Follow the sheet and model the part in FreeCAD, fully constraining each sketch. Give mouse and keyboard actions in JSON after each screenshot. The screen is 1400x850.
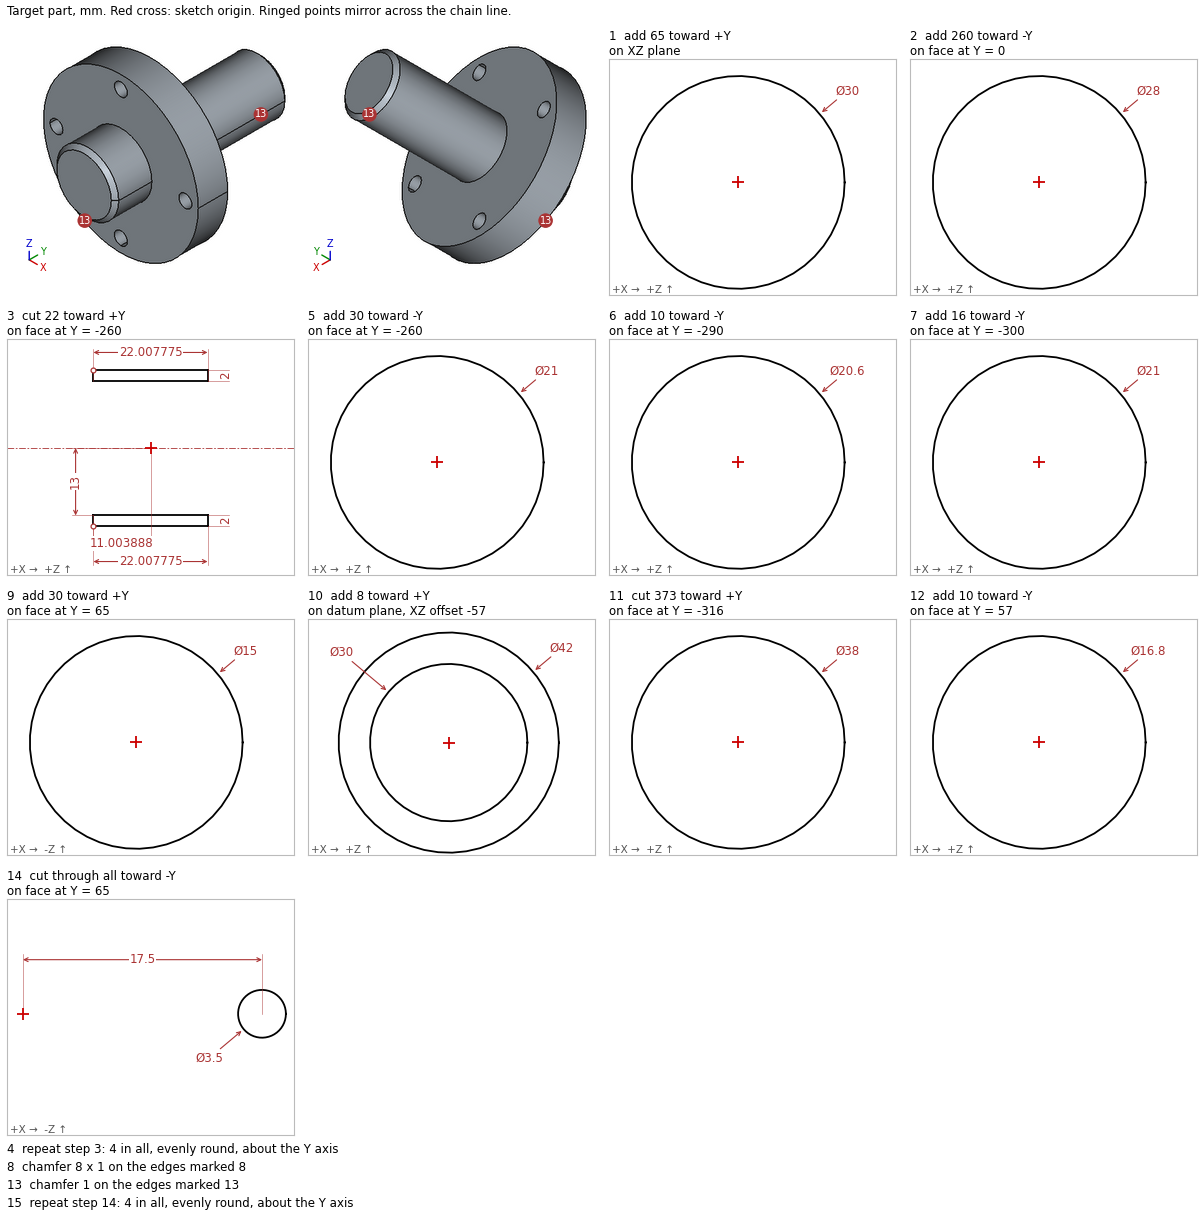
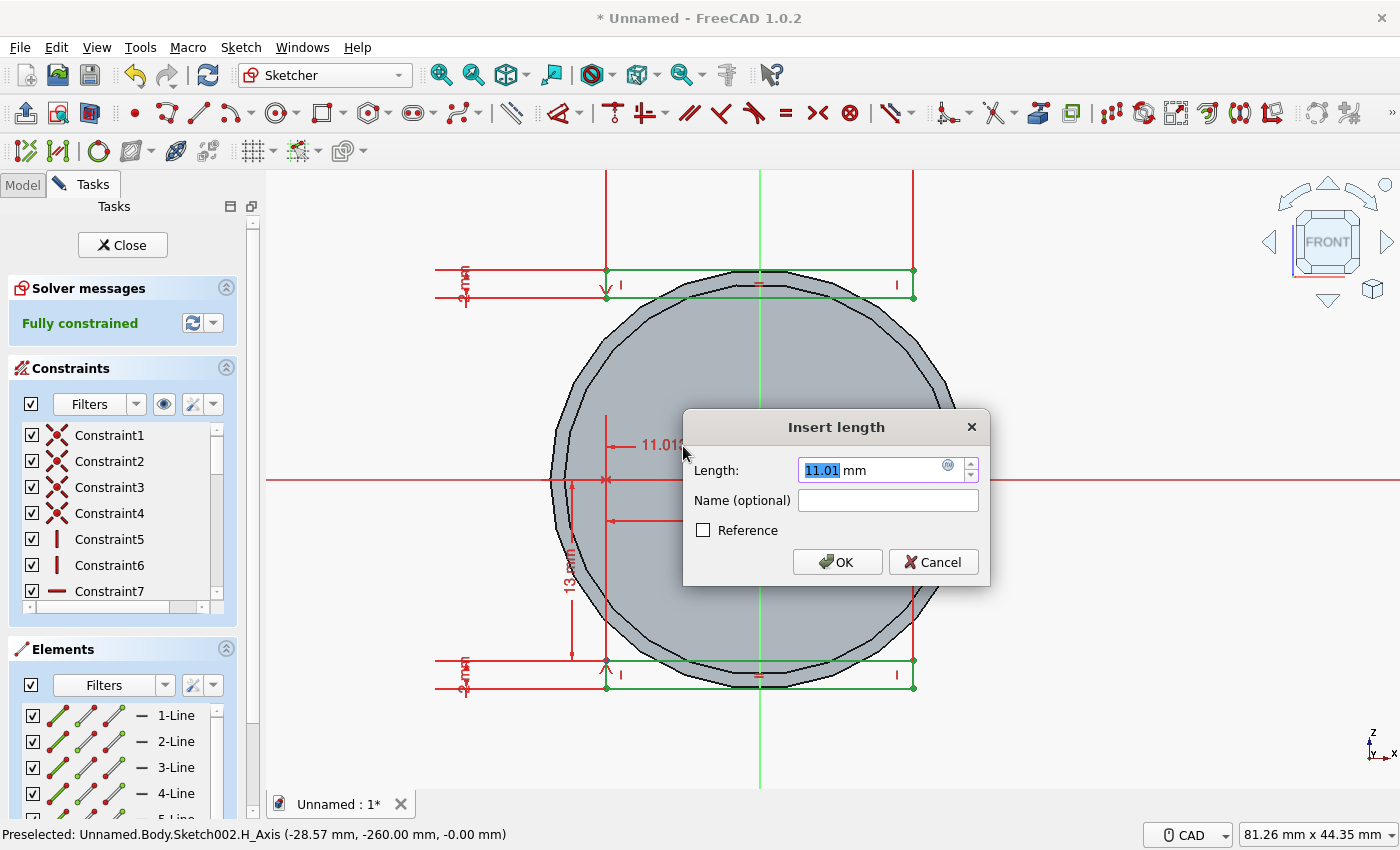
{"action": "type", "text": "11.003888"}
{"action": "key", "text": "Return"}
{"action": "key", "text": "Escape"}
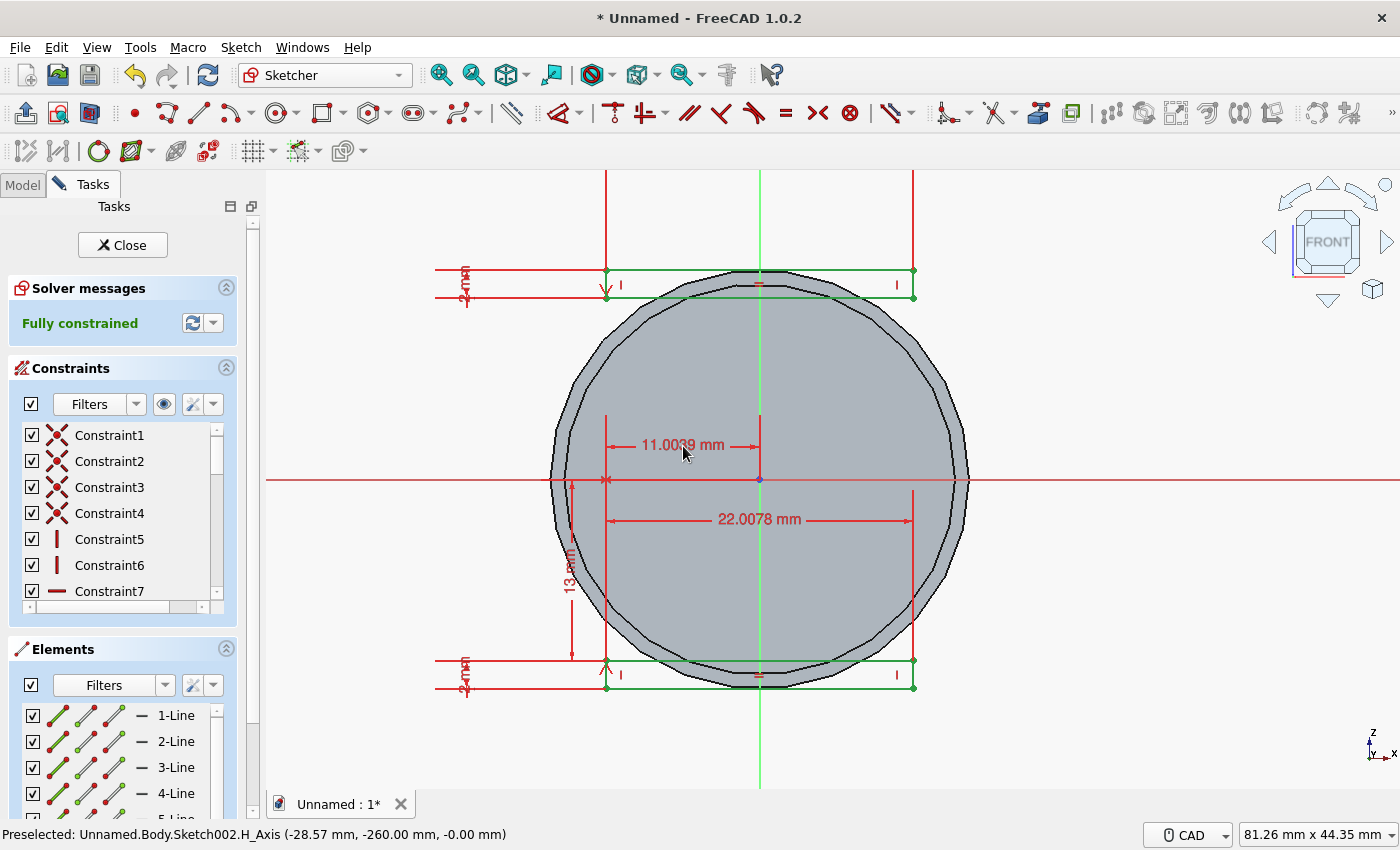
{"action": "left_click", "coordinate": [123, 245]}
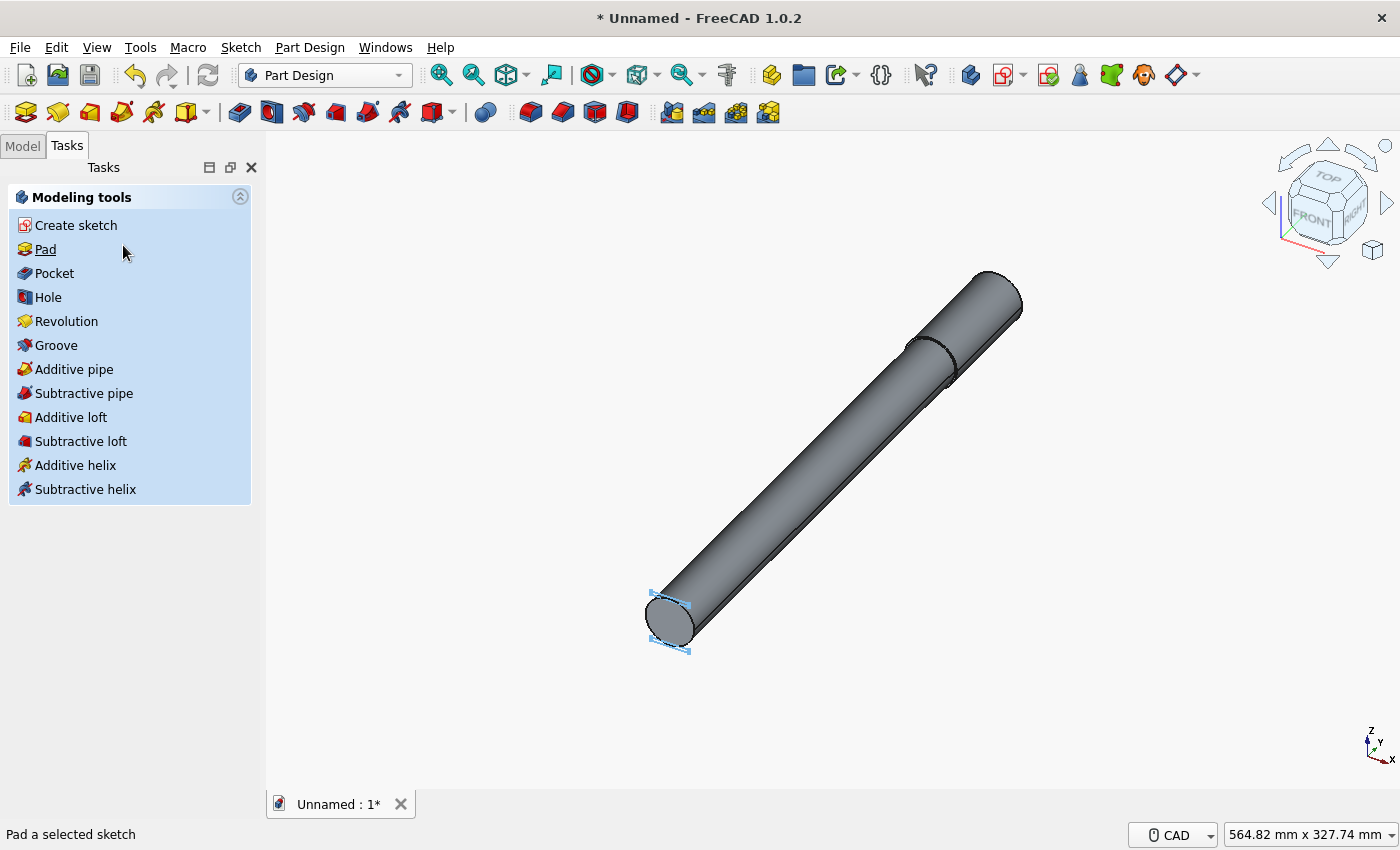
{"action": "left_click", "coordinate": [240, 112]}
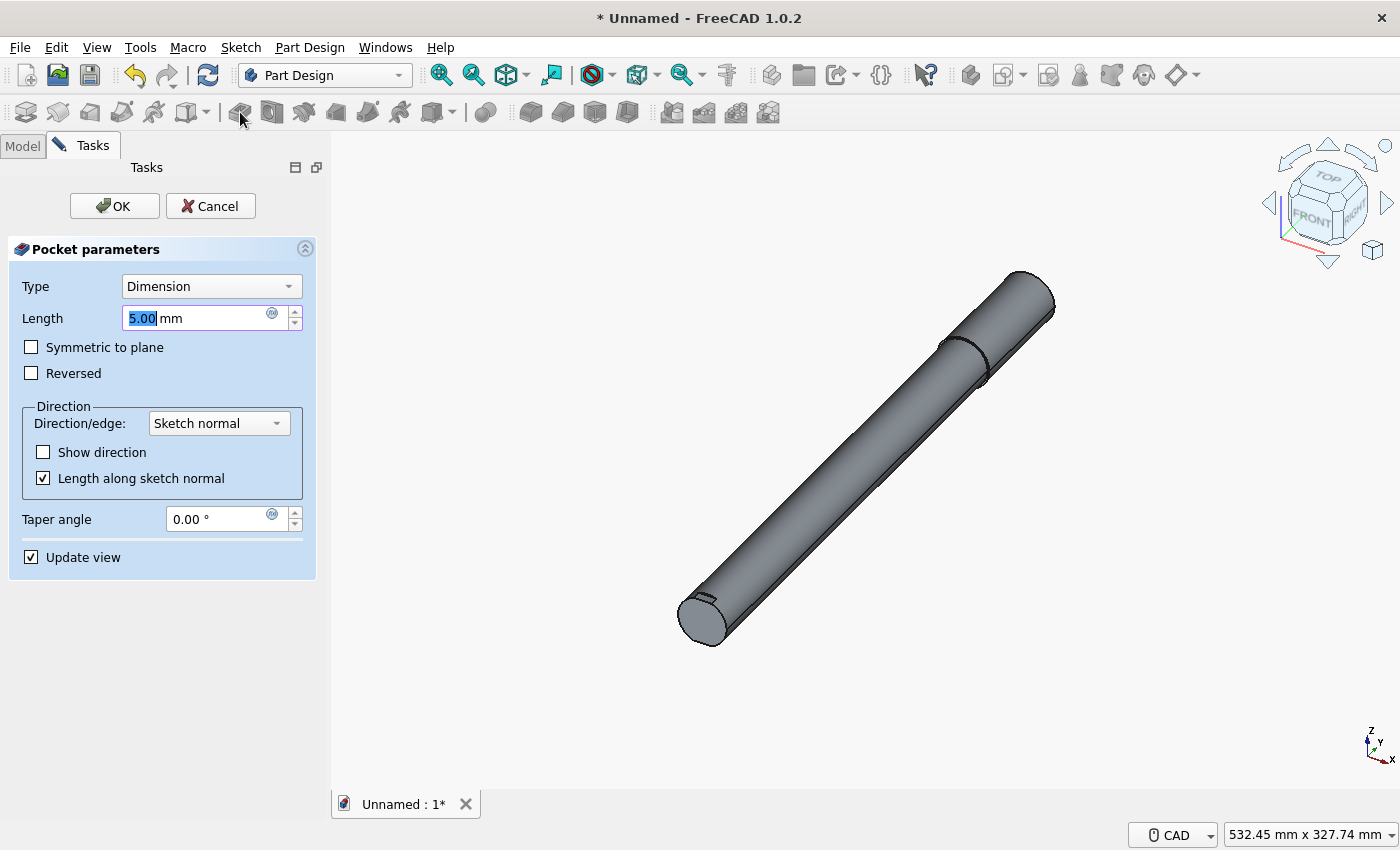
{"action": "type", "text": "22"}
{"action": "key", "text": "Tab"}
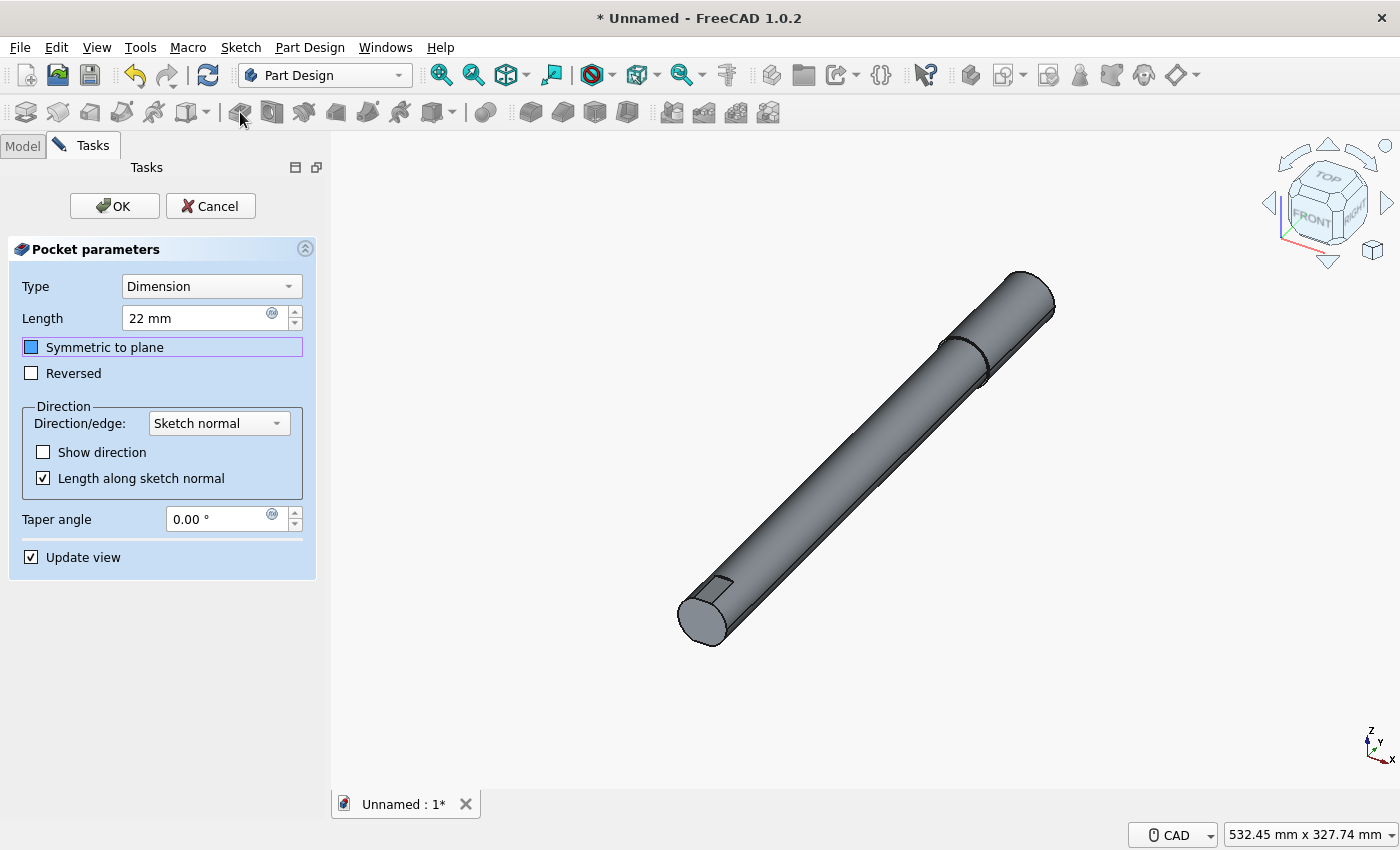
{"action": "left_click", "coordinate": [115, 206]}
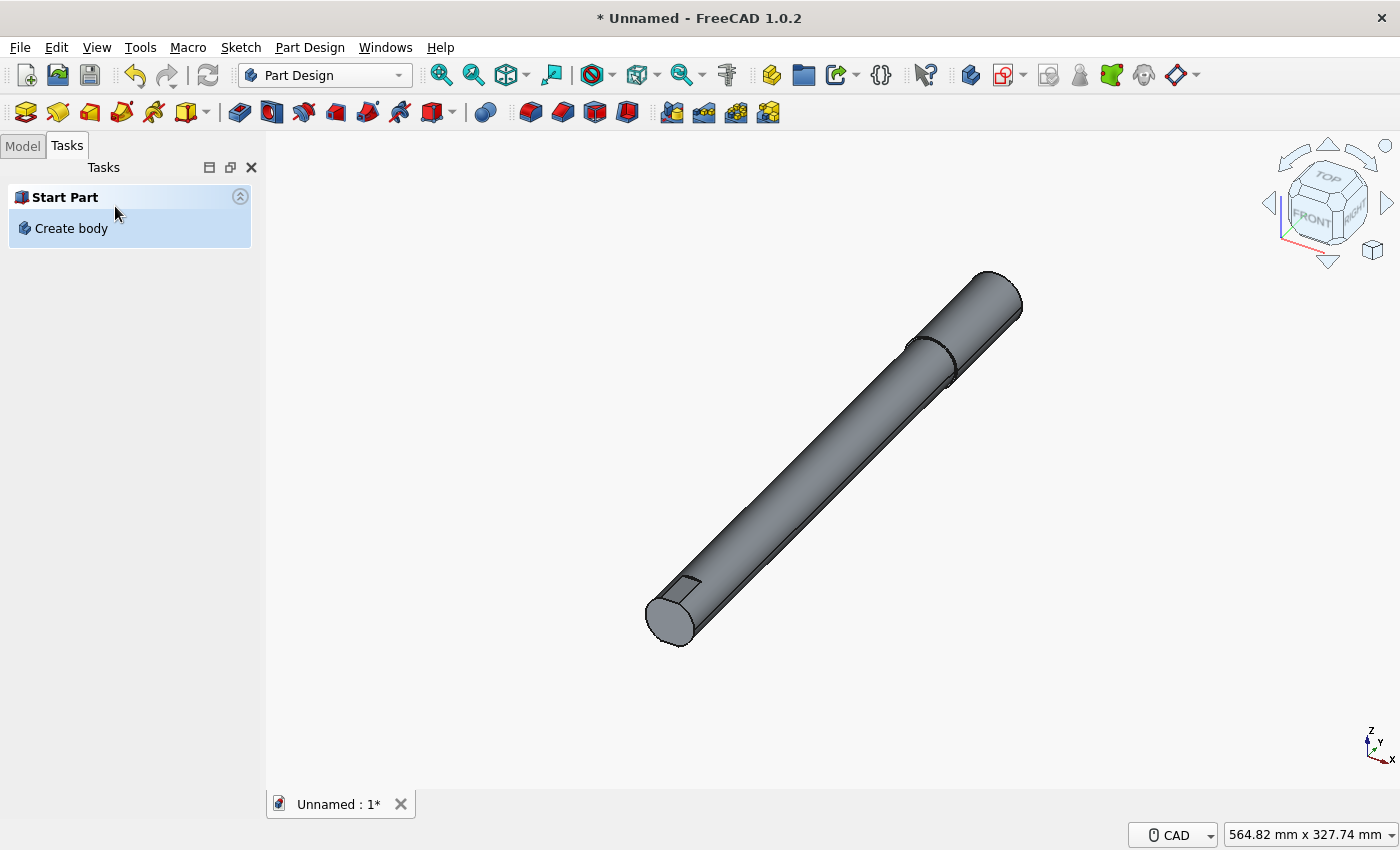
{"action": "left_click", "coordinate": [23, 145]}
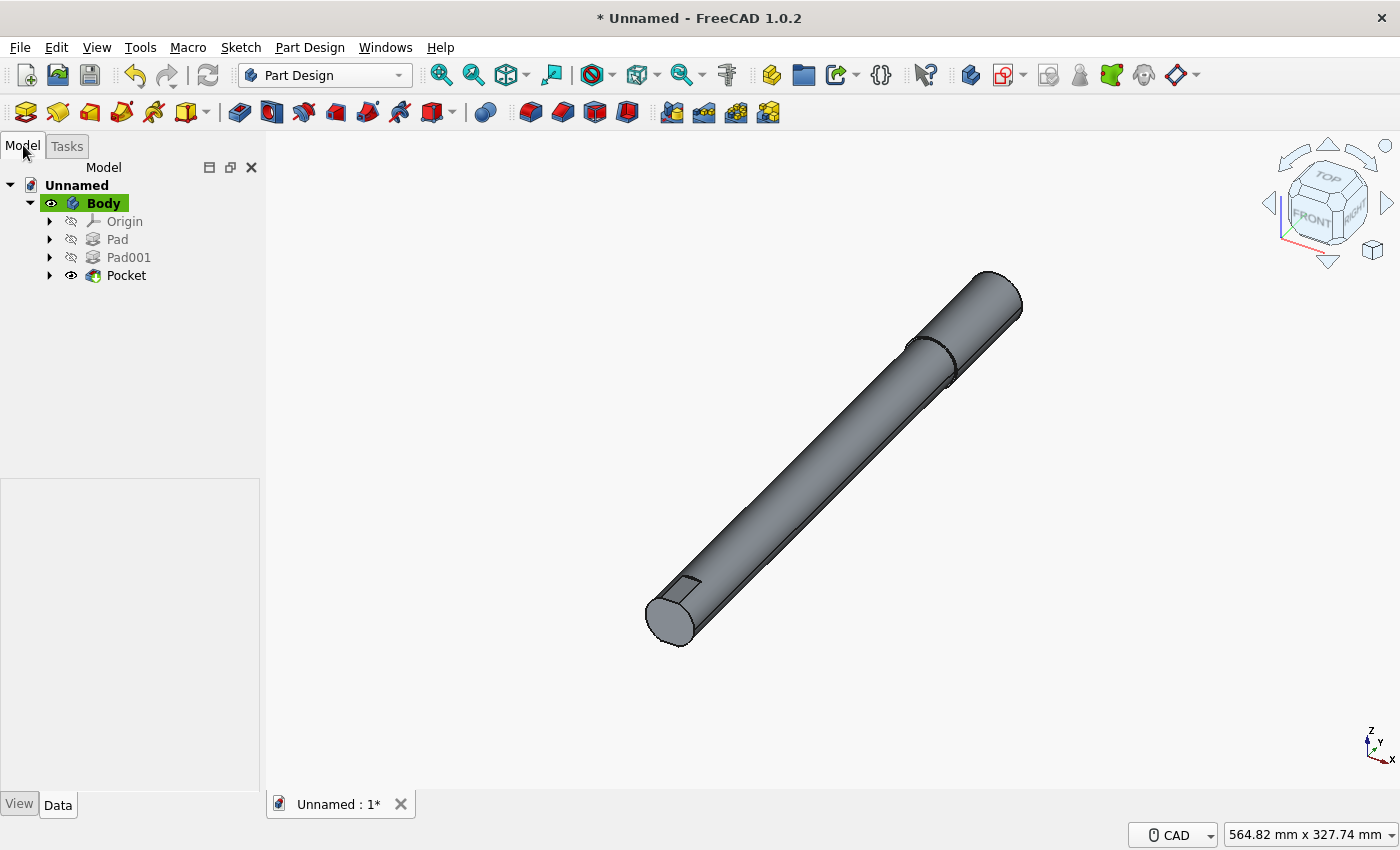
{"action": "left_click", "coordinate": [116, 275]}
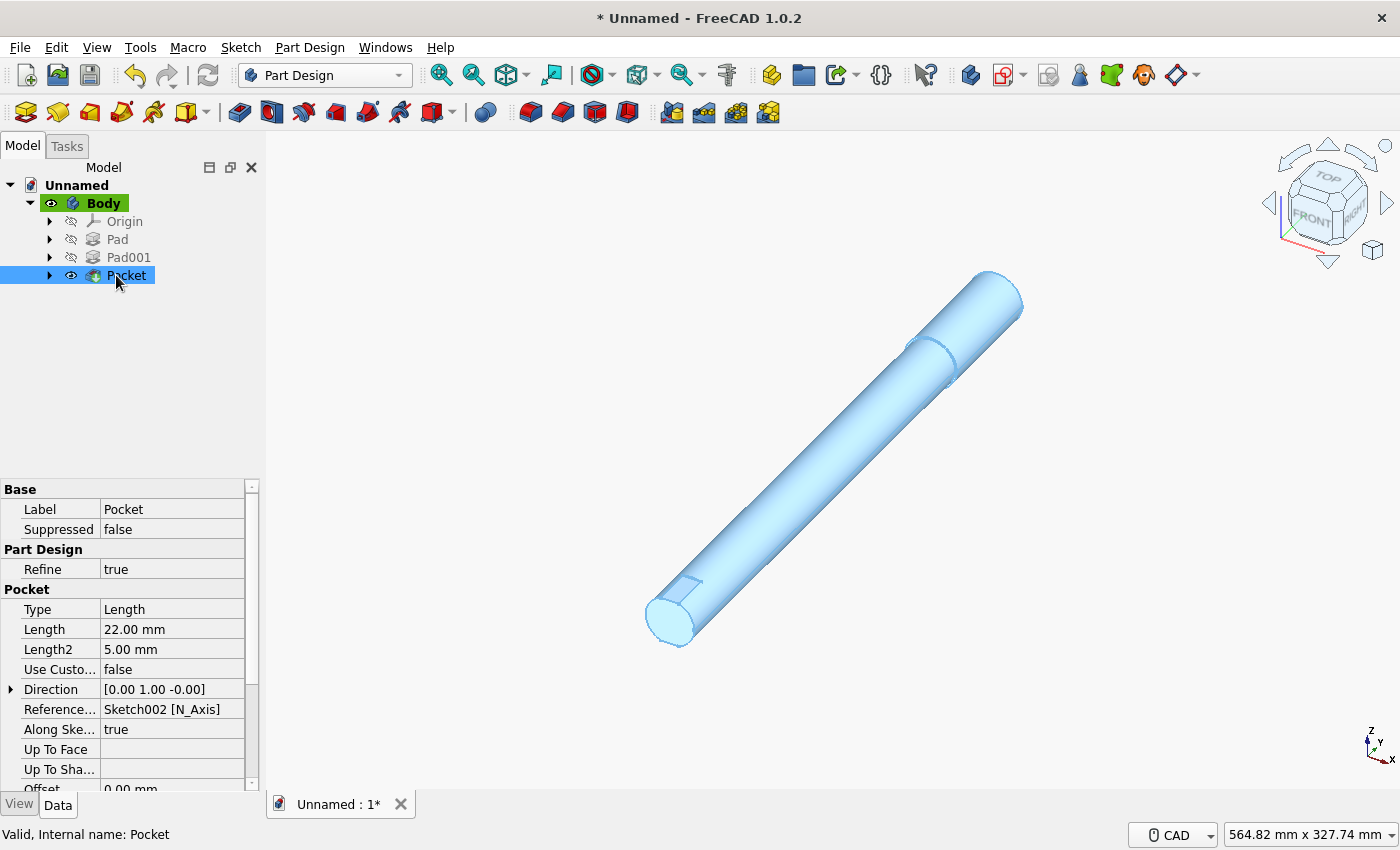
{"action": "left_click", "coordinate": [736, 112]}